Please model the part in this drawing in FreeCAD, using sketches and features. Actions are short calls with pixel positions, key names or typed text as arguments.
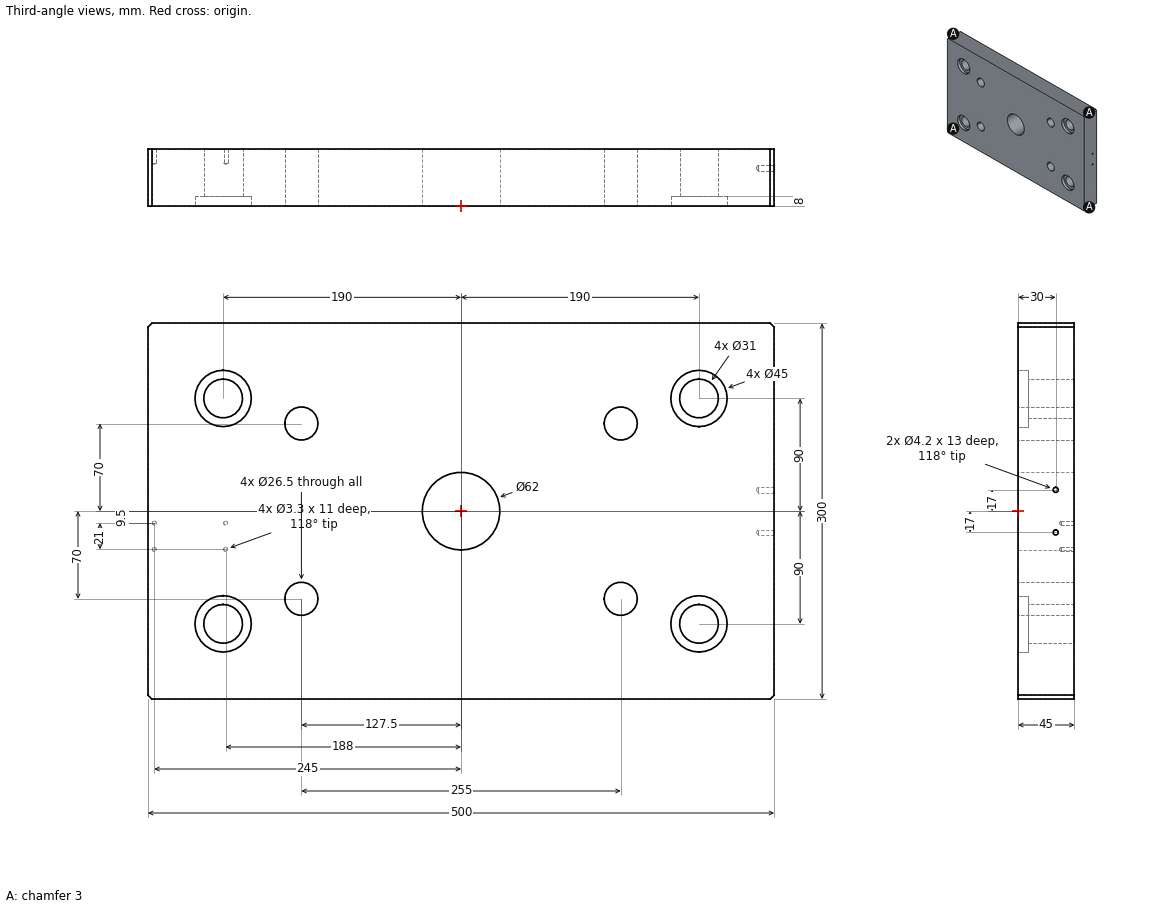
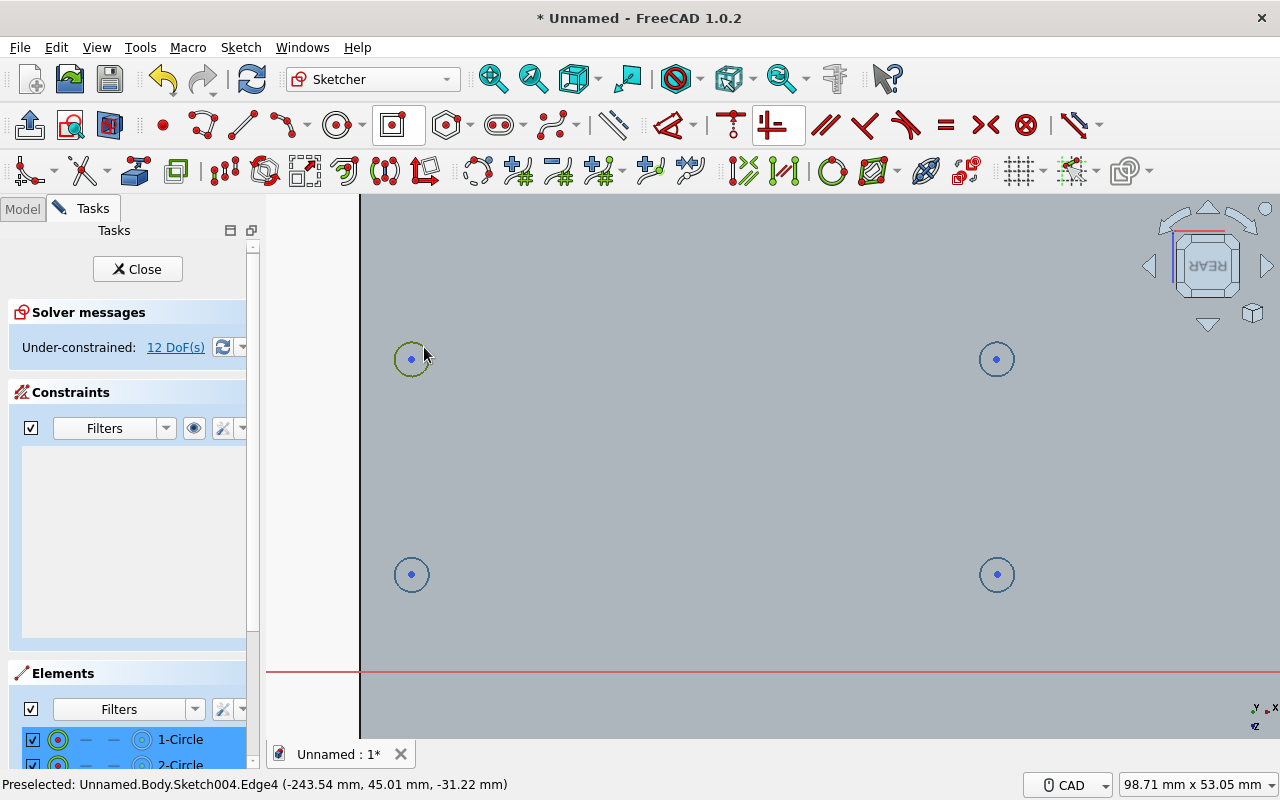
key(e)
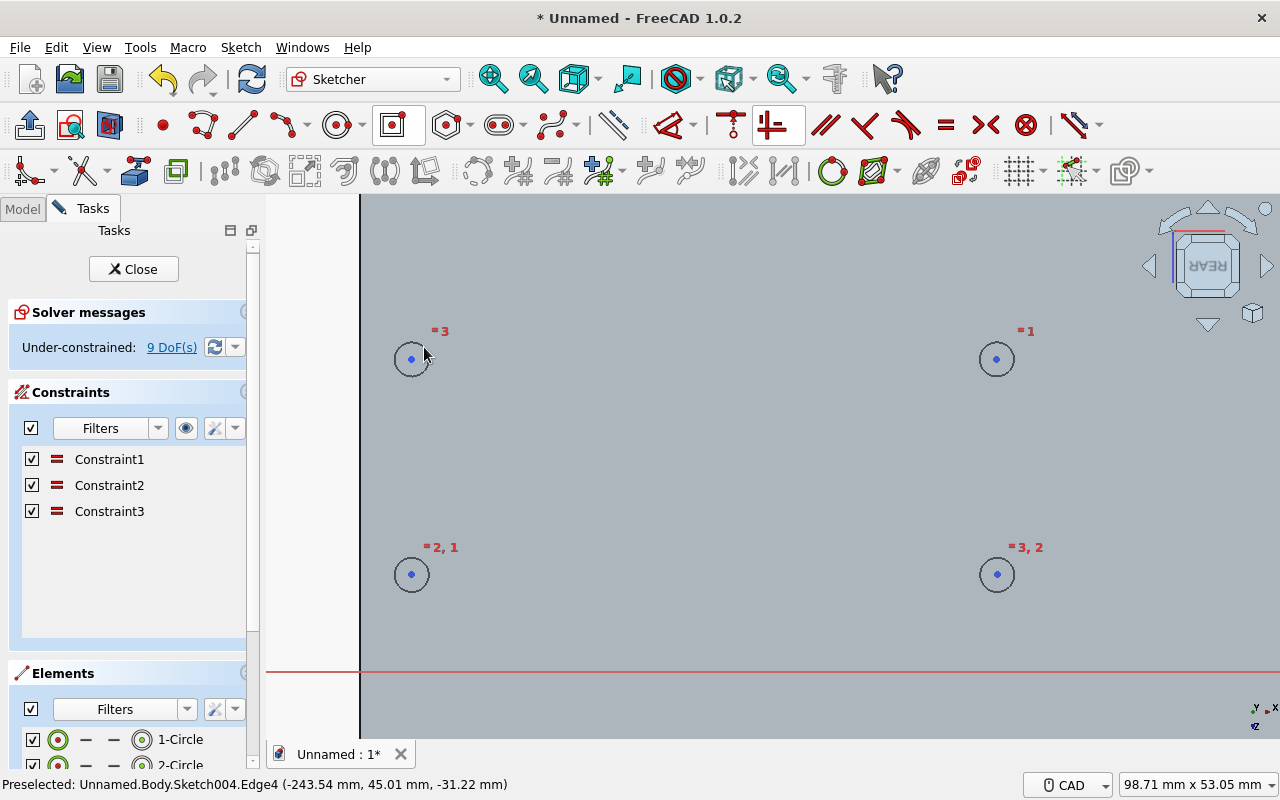
click(997, 359)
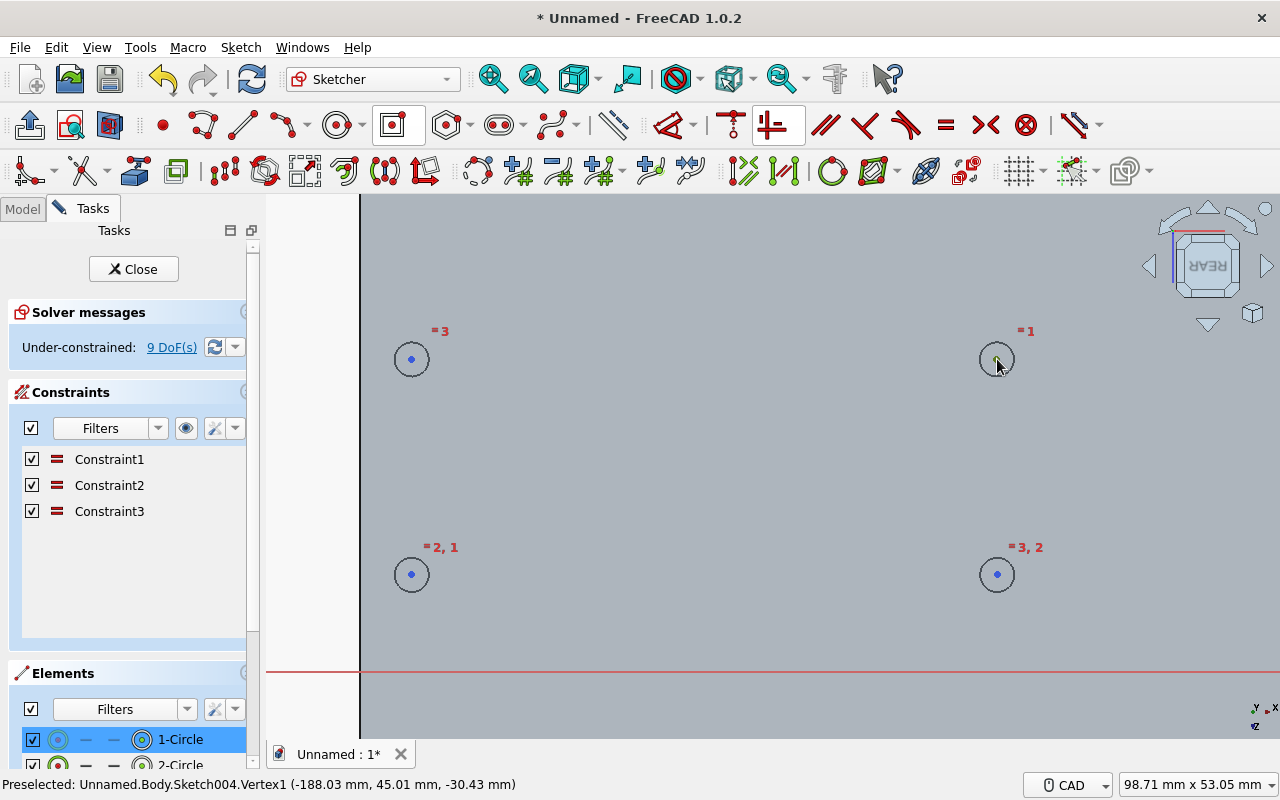
click(997, 575)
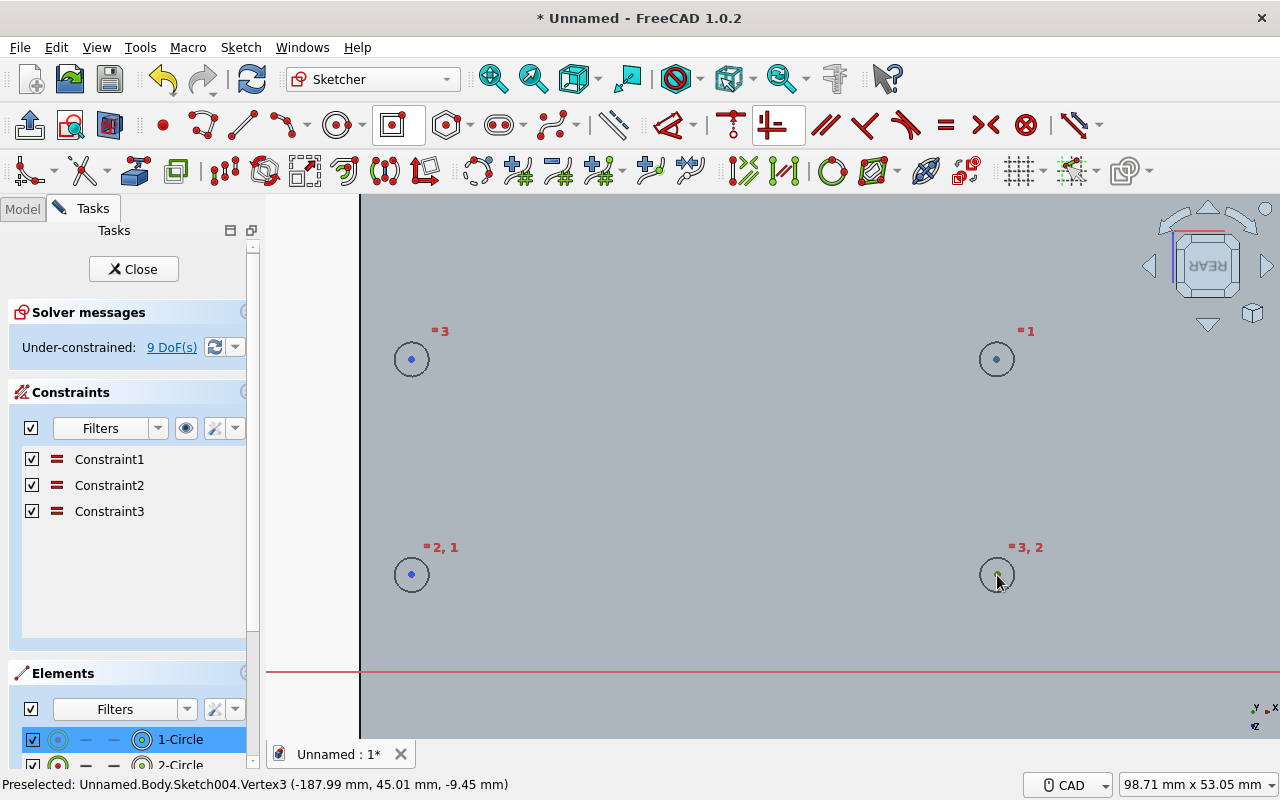
key(v)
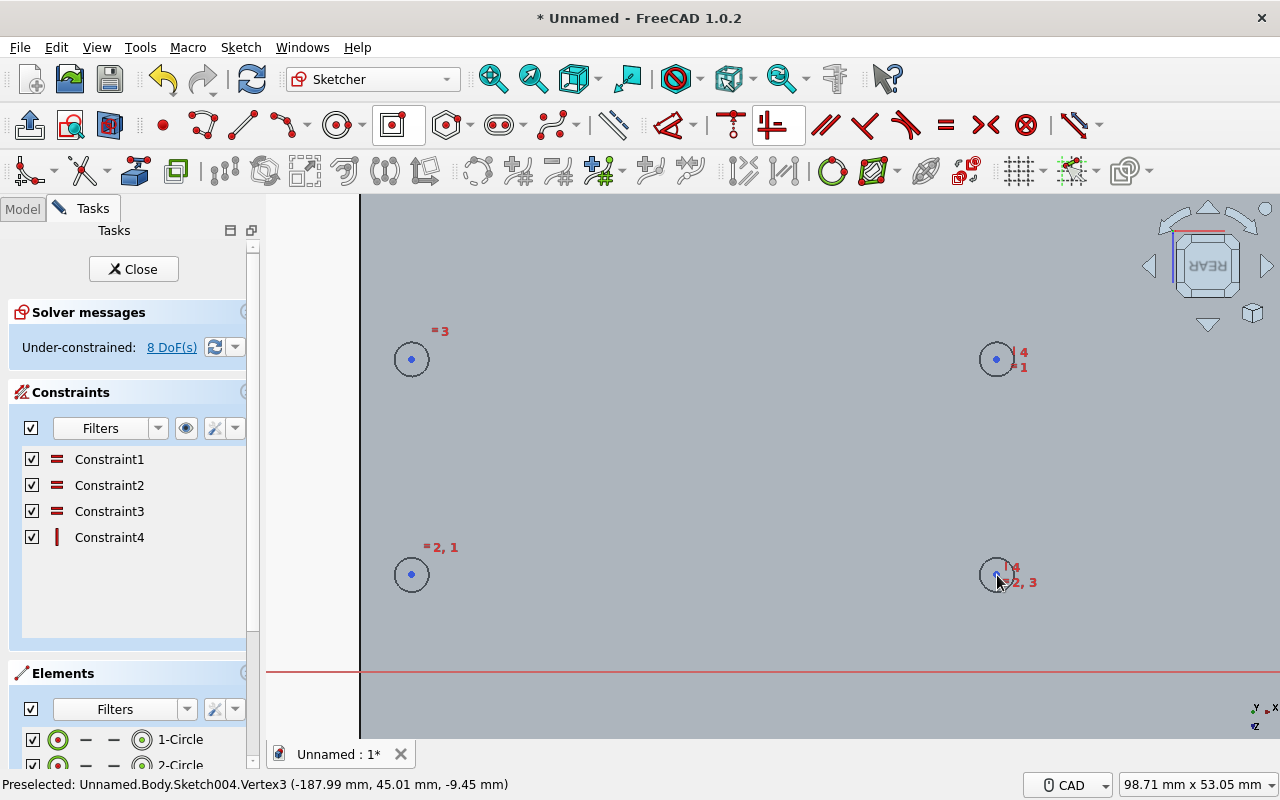
click(412, 575)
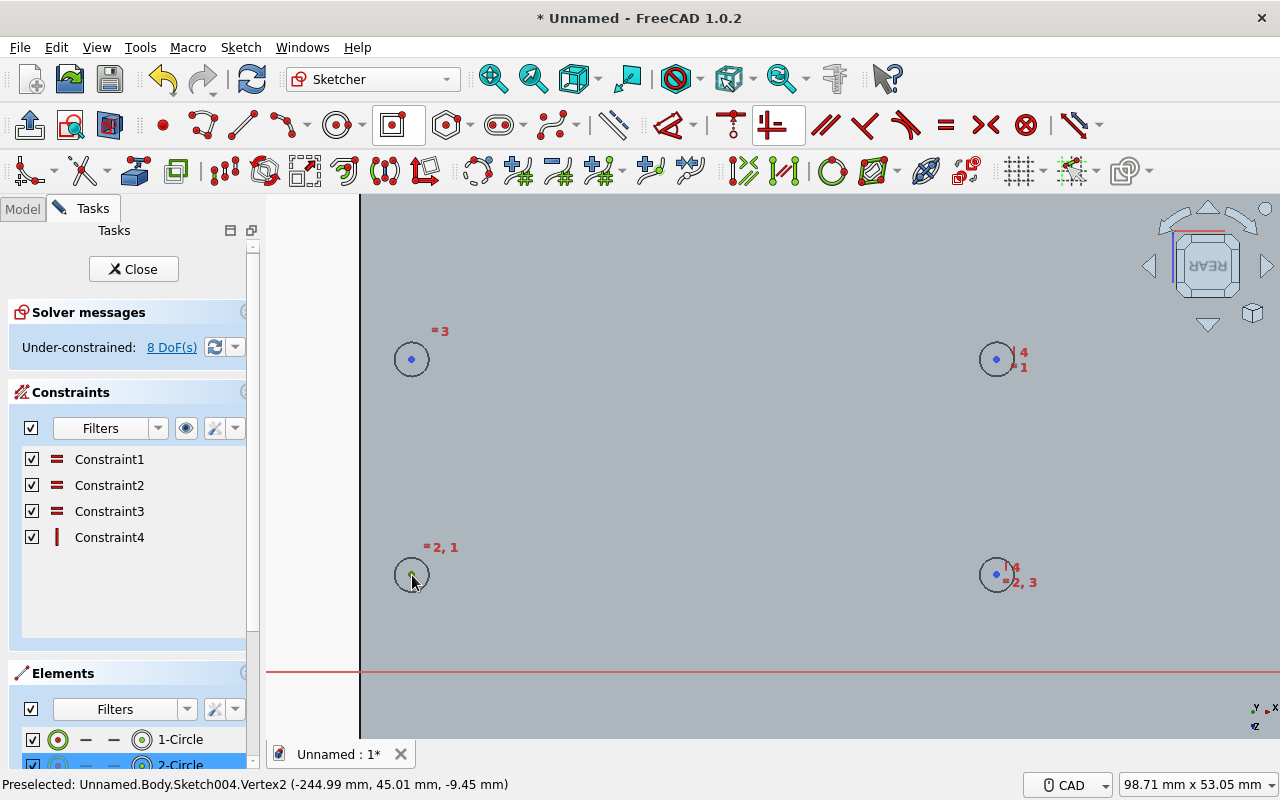
click(997, 575)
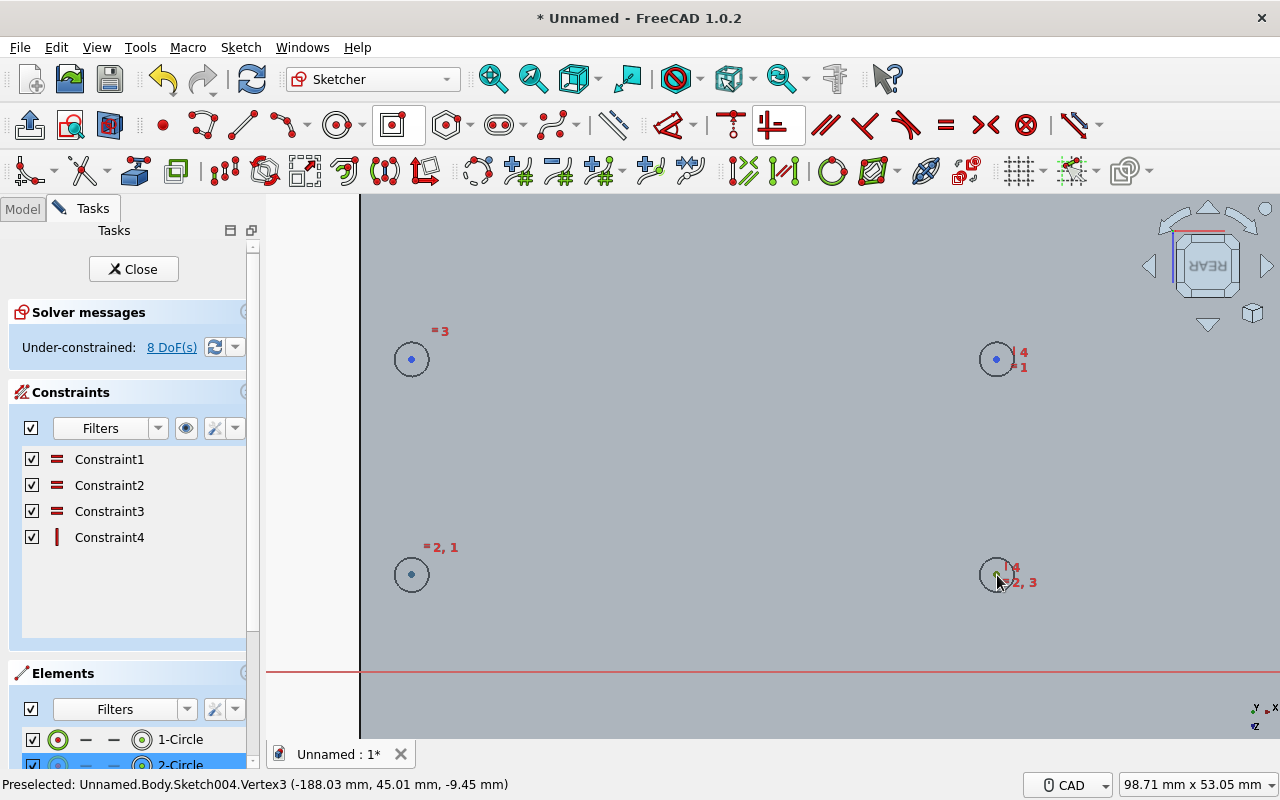
key(h)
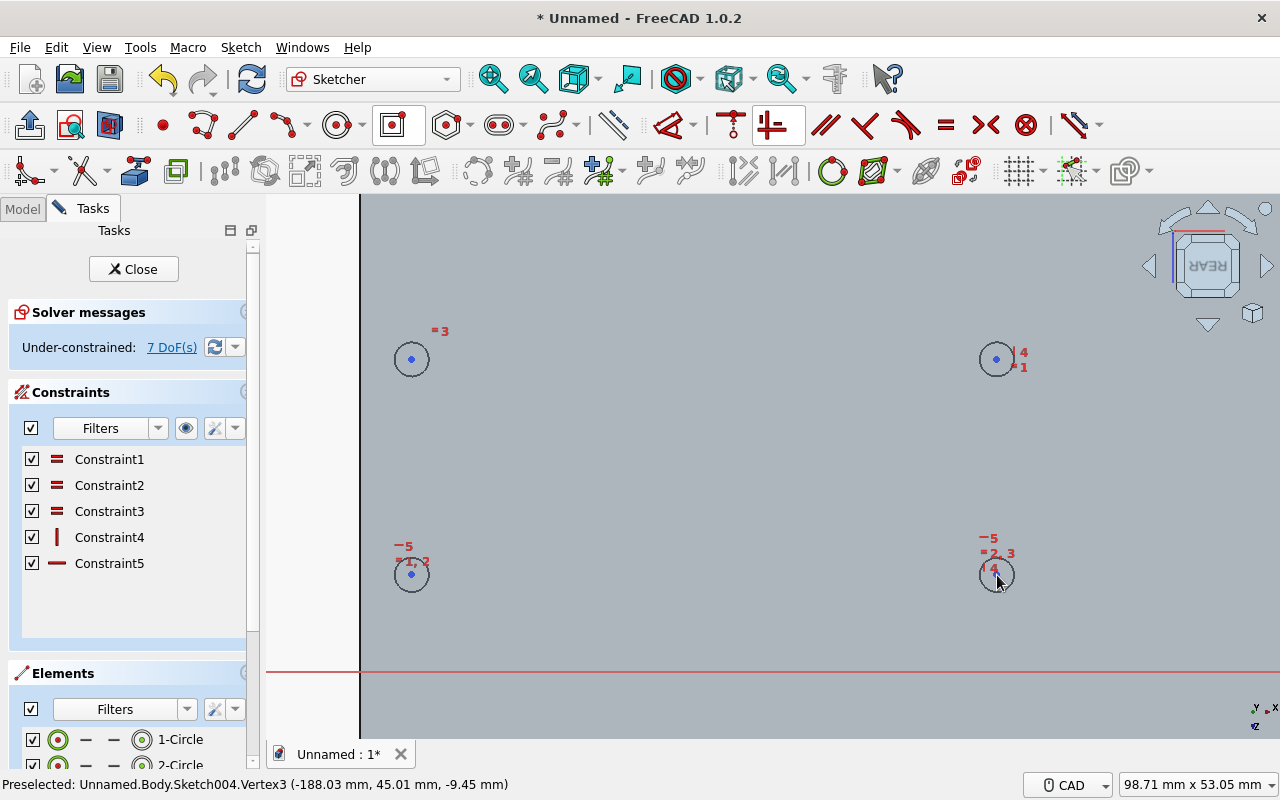
click(412, 575)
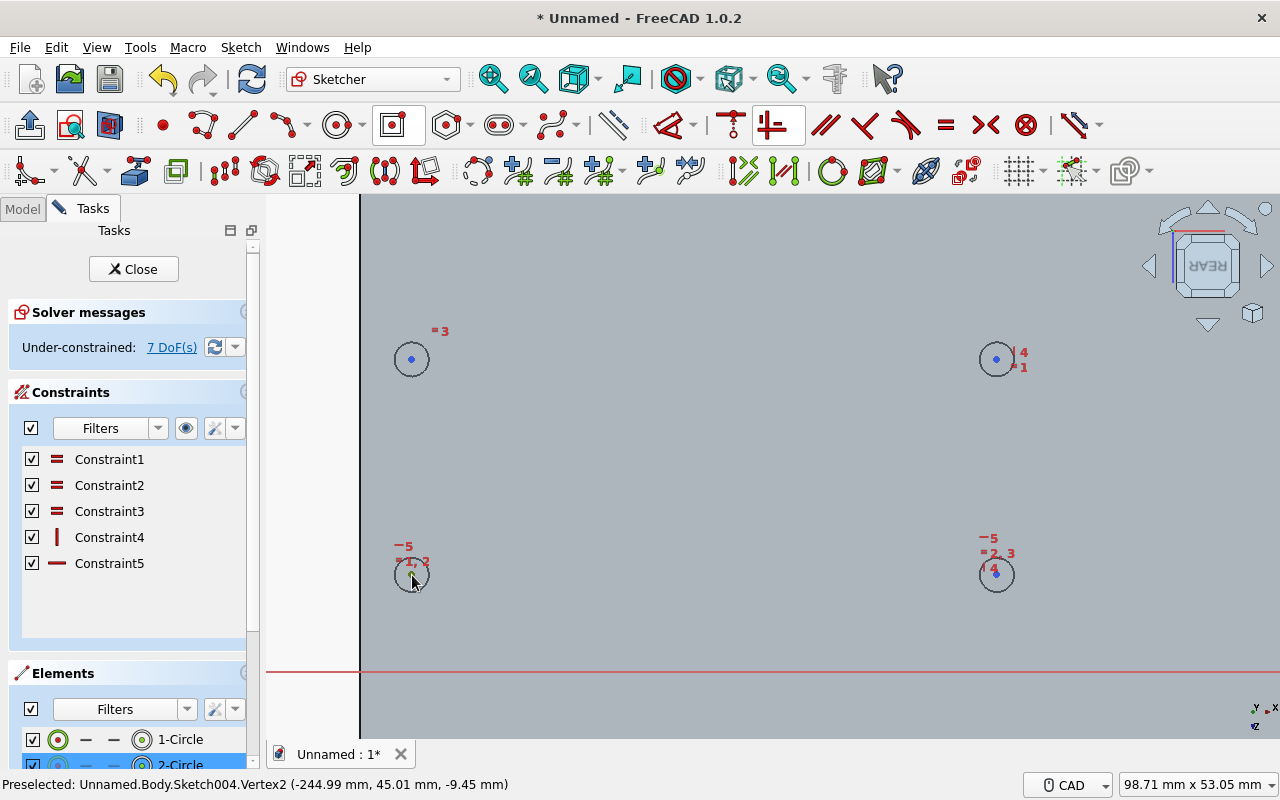
click(412, 359)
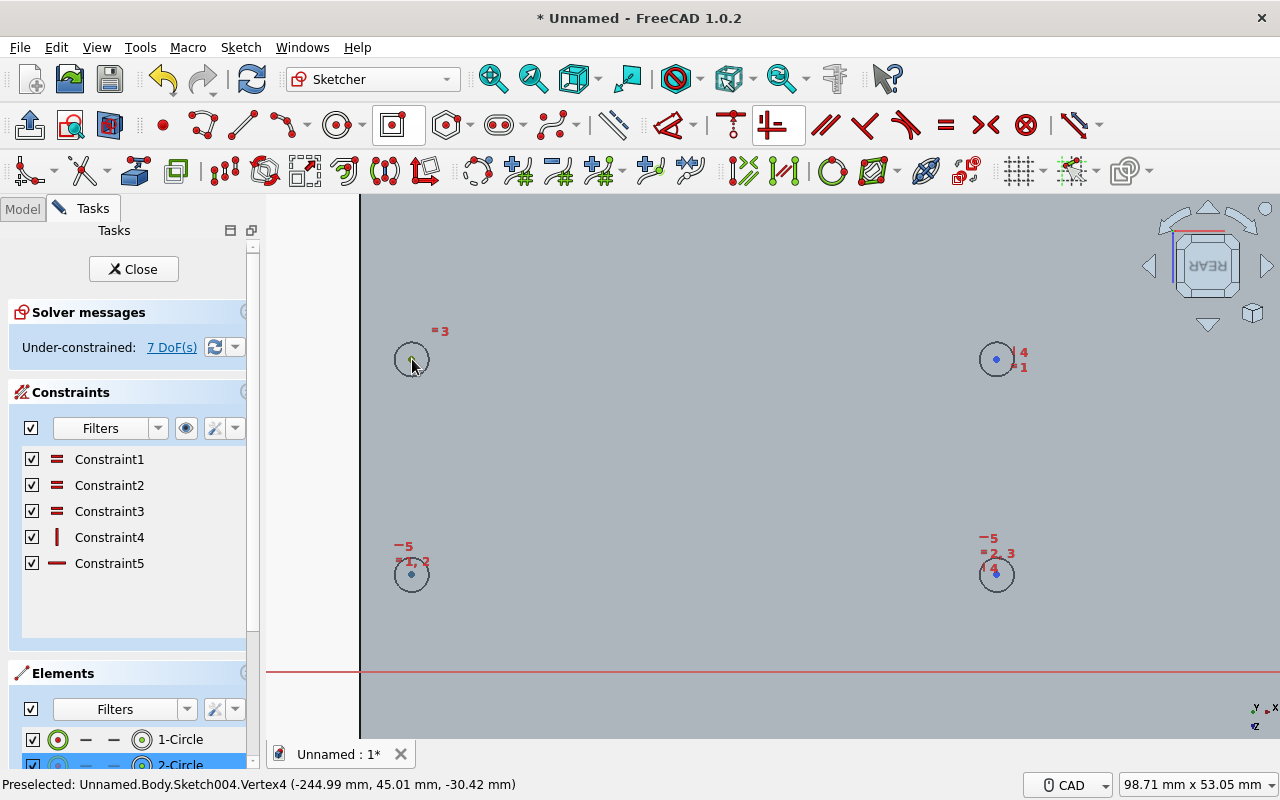
key(v)